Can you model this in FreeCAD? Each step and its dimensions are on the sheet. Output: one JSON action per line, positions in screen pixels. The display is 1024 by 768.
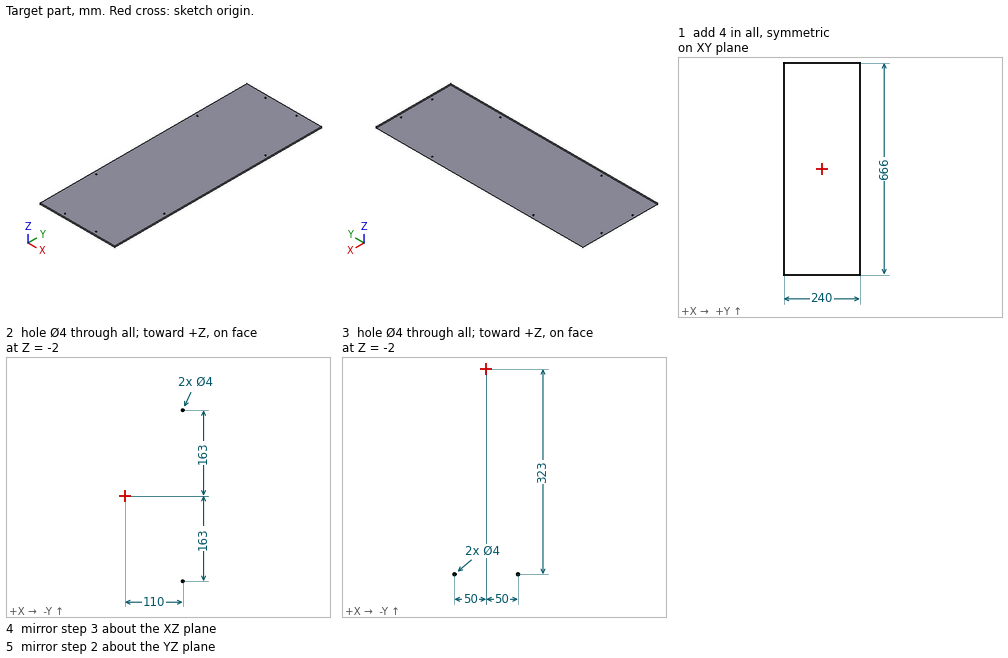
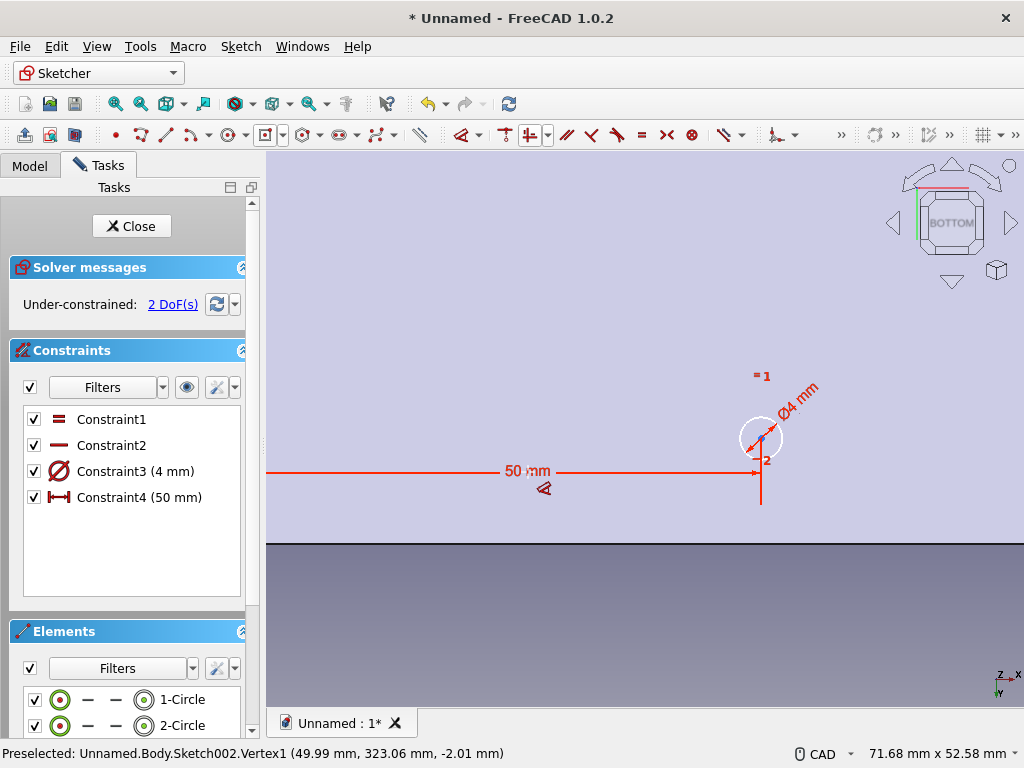
{"action": "scroll", "coordinate": [777, 424], "scroll_direction": "down", "scroll_amount": 5}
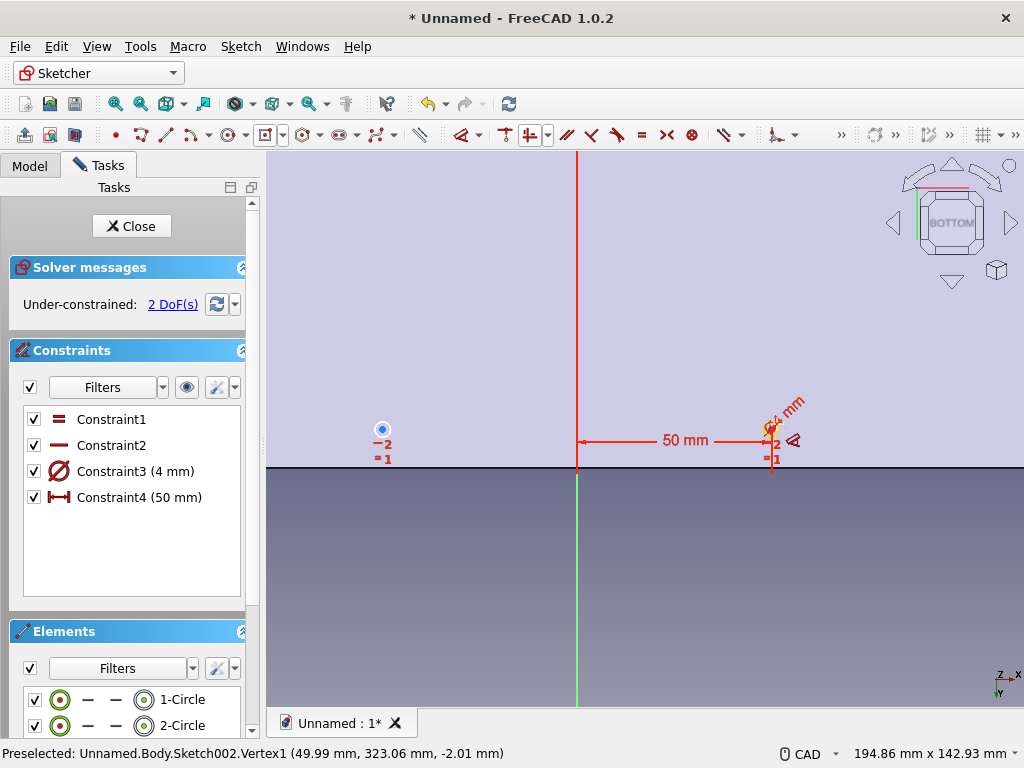
{"action": "left_click", "coordinate": [383, 430]}
{"action": "left_click", "coordinate": [480, 464]}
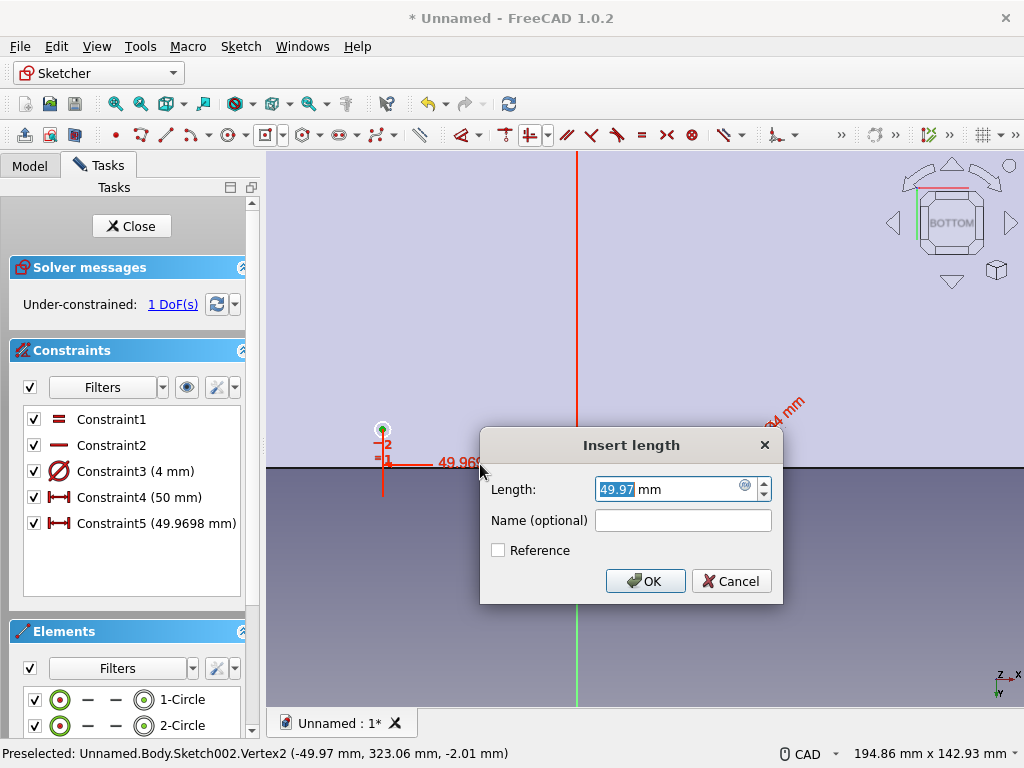
{"action": "type", "text": "50"}
{"action": "key", "text": "Return"}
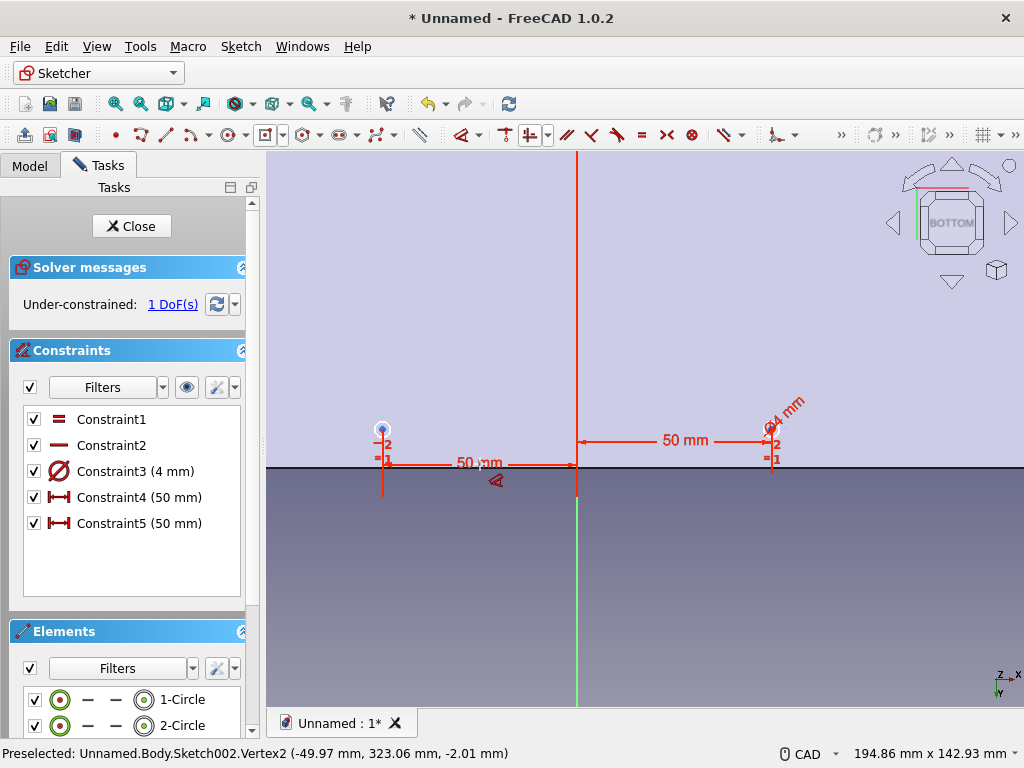
{"action": "left_click", "coordinate": [772, 430]}
{"action": "left_click", "coordinate": [806, 304]}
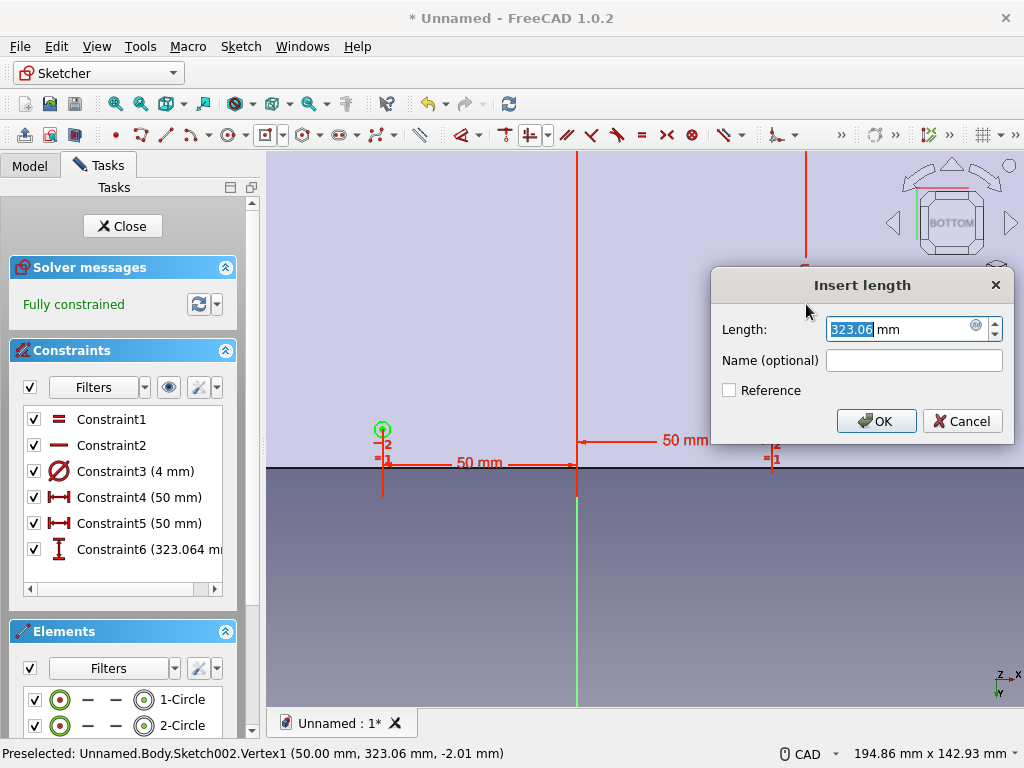
{"action": "type", "text": "323"}
{"action": "key", "text": "Return"}
{"action": "key", "text": "Escape"}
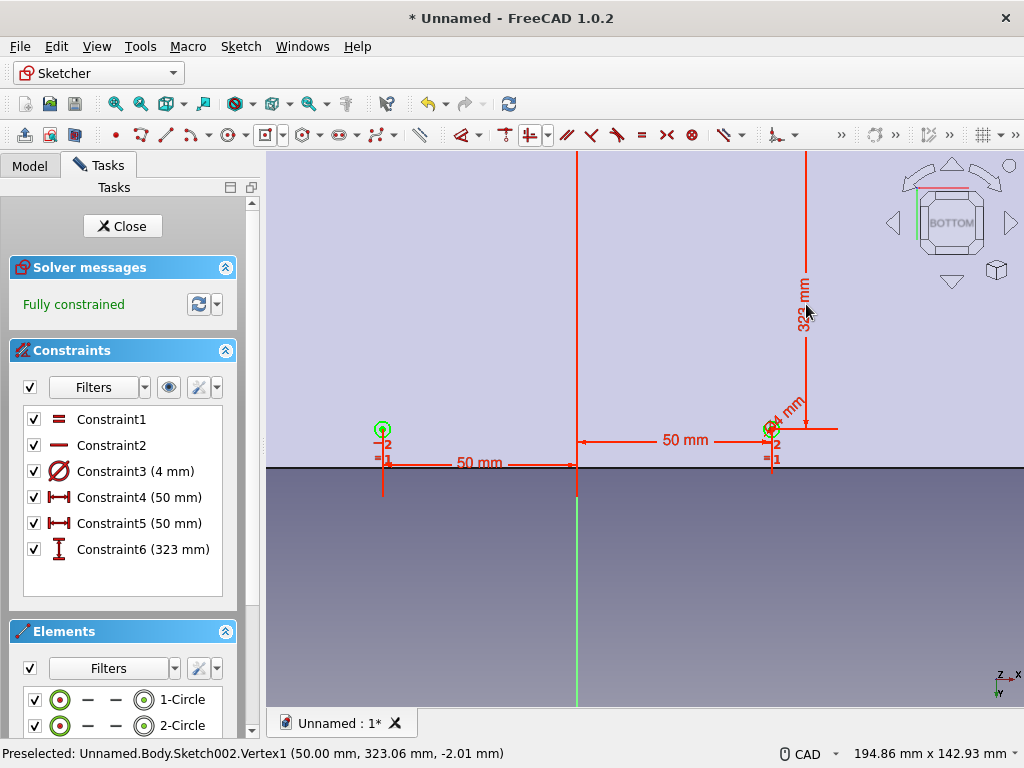
{"action": "left_click", "coordinate": [123, 226]}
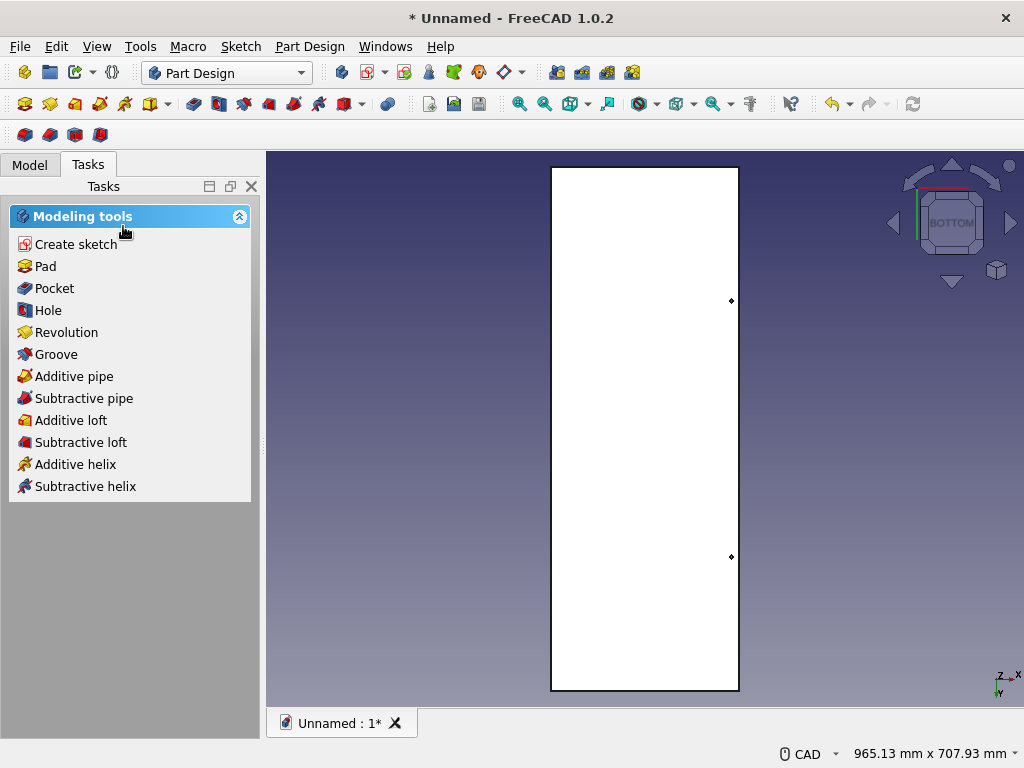
{"action": "left_click", "coordinate": [219, 104]}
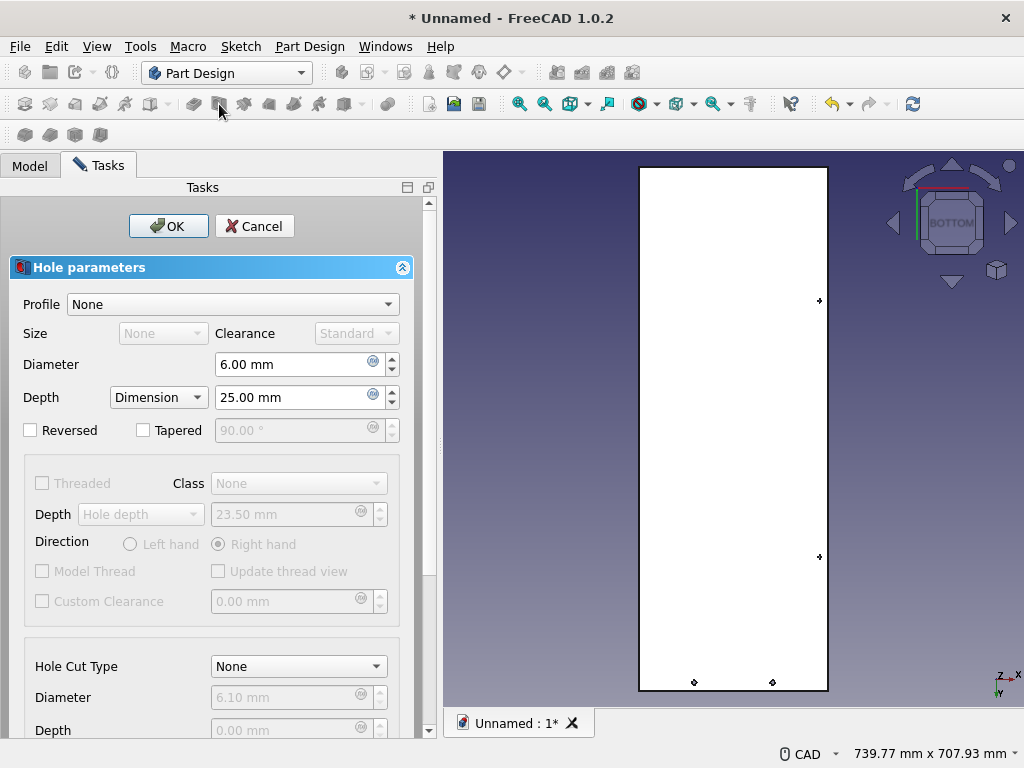
{"action": "triple_click", "coordinate": [300, 364]}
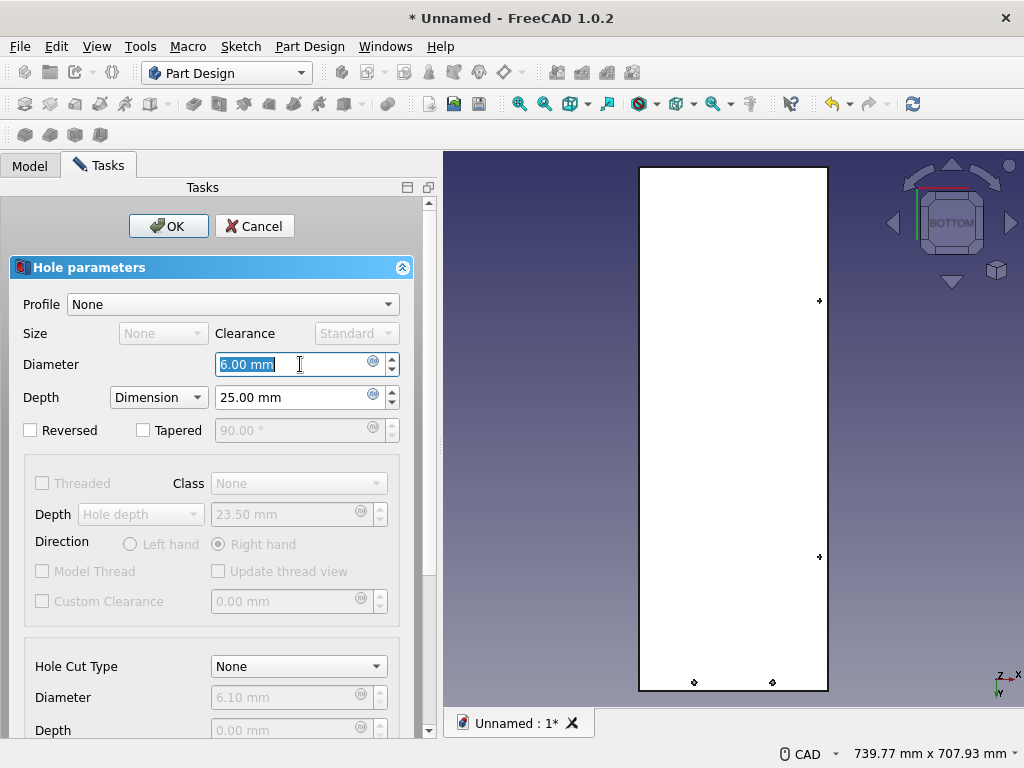
{"action": "type", "text": "4"}
{"action": "key", "text": "Tab"}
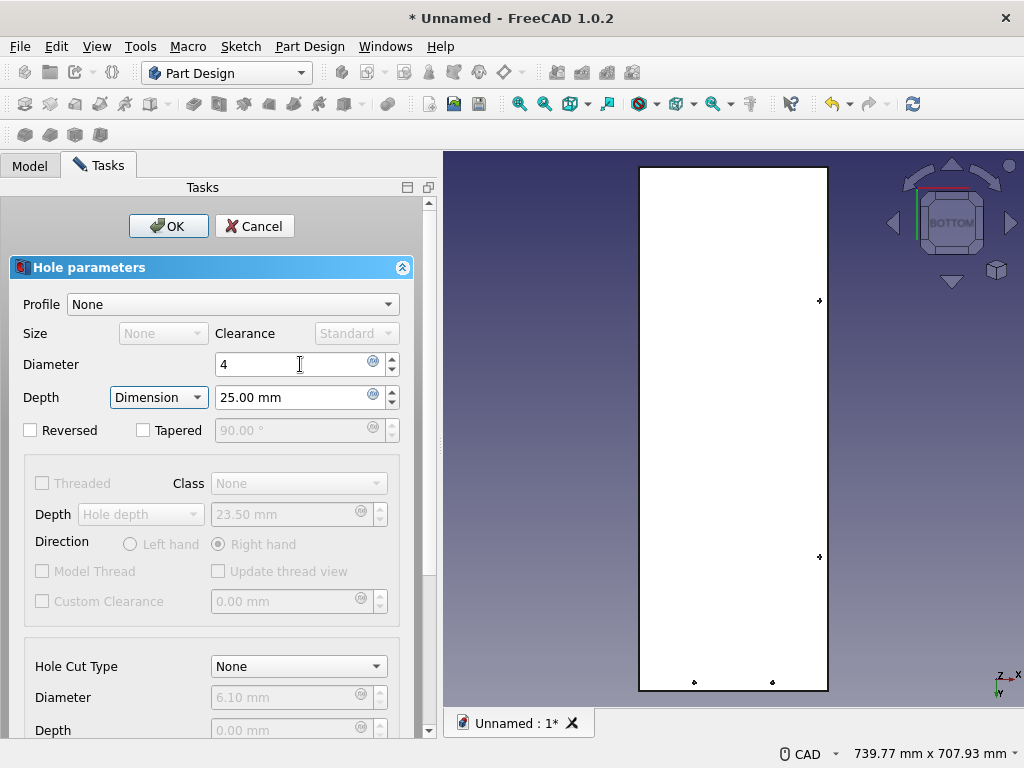
{"action": "left_click", "coordinate": [160, 398]}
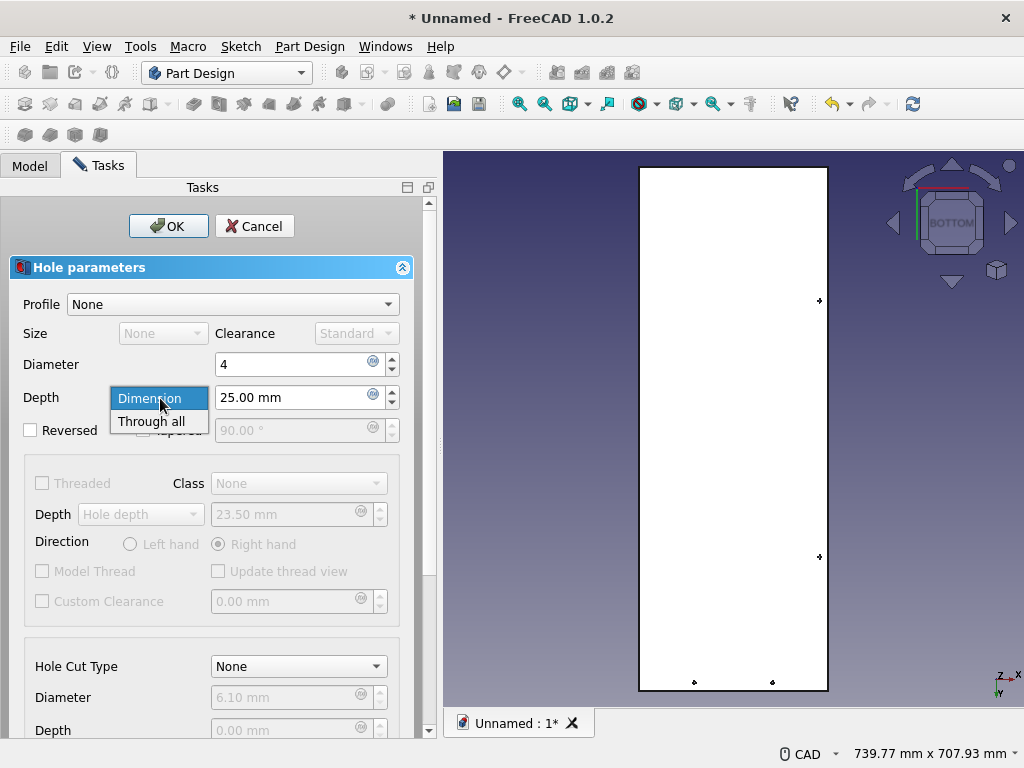
{"action": "left_click", "coordinate": [158, 422]}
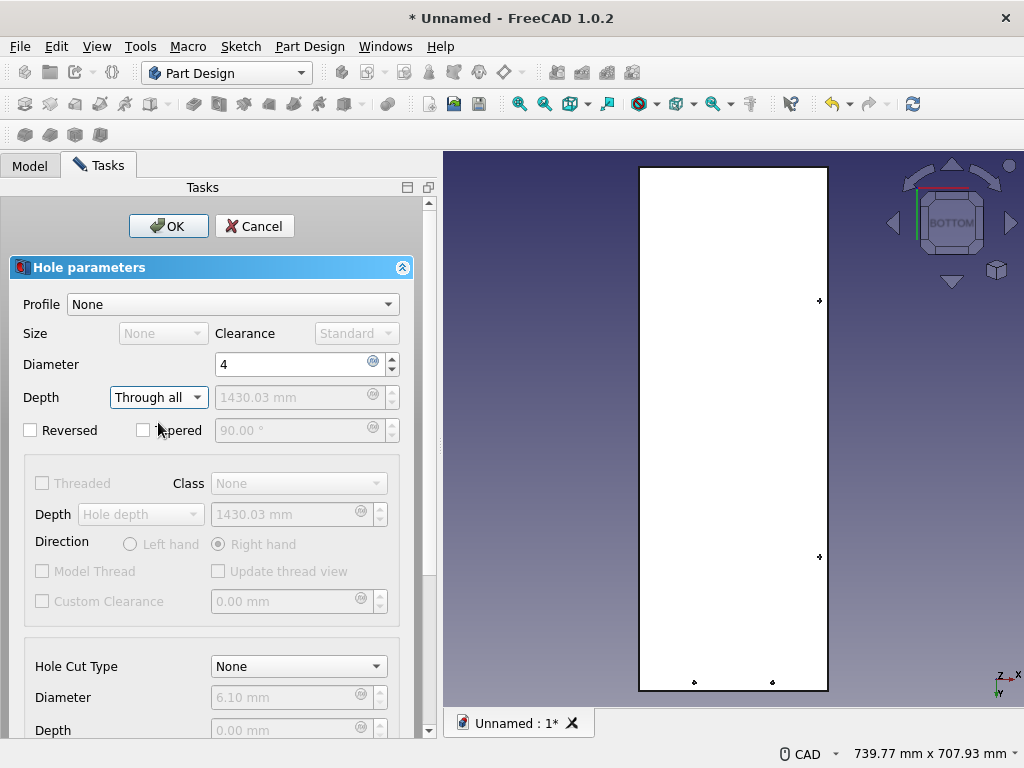
{"action": "left_click", "coordinate": [169, 226]}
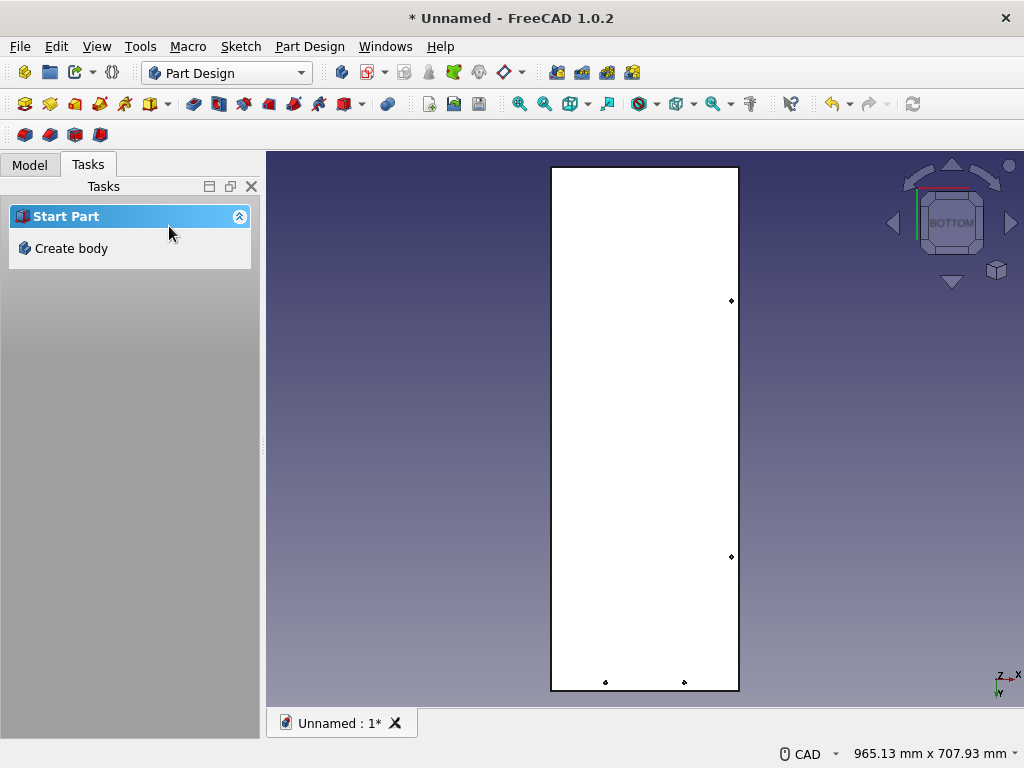
{"action": "left_click", "coordinate": [30, 164]}